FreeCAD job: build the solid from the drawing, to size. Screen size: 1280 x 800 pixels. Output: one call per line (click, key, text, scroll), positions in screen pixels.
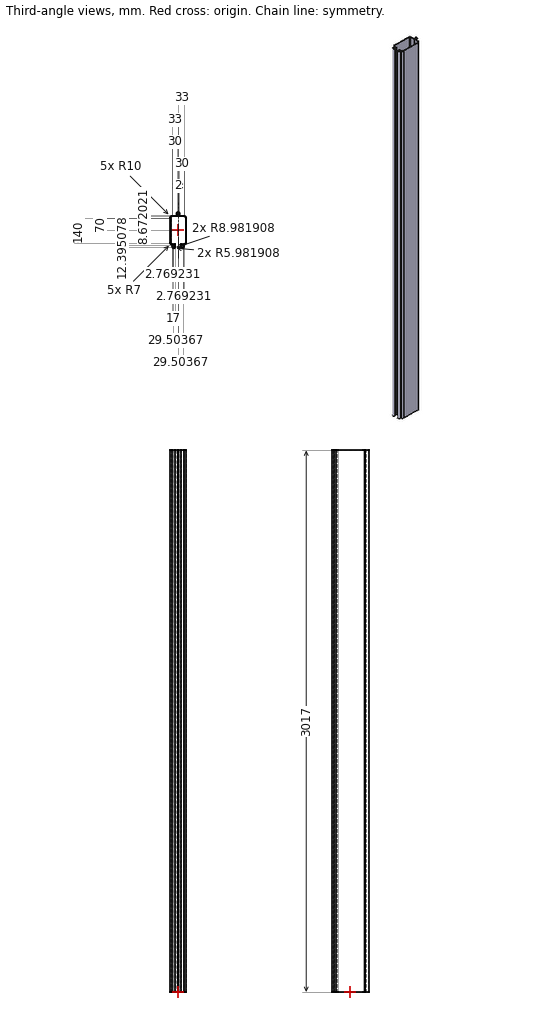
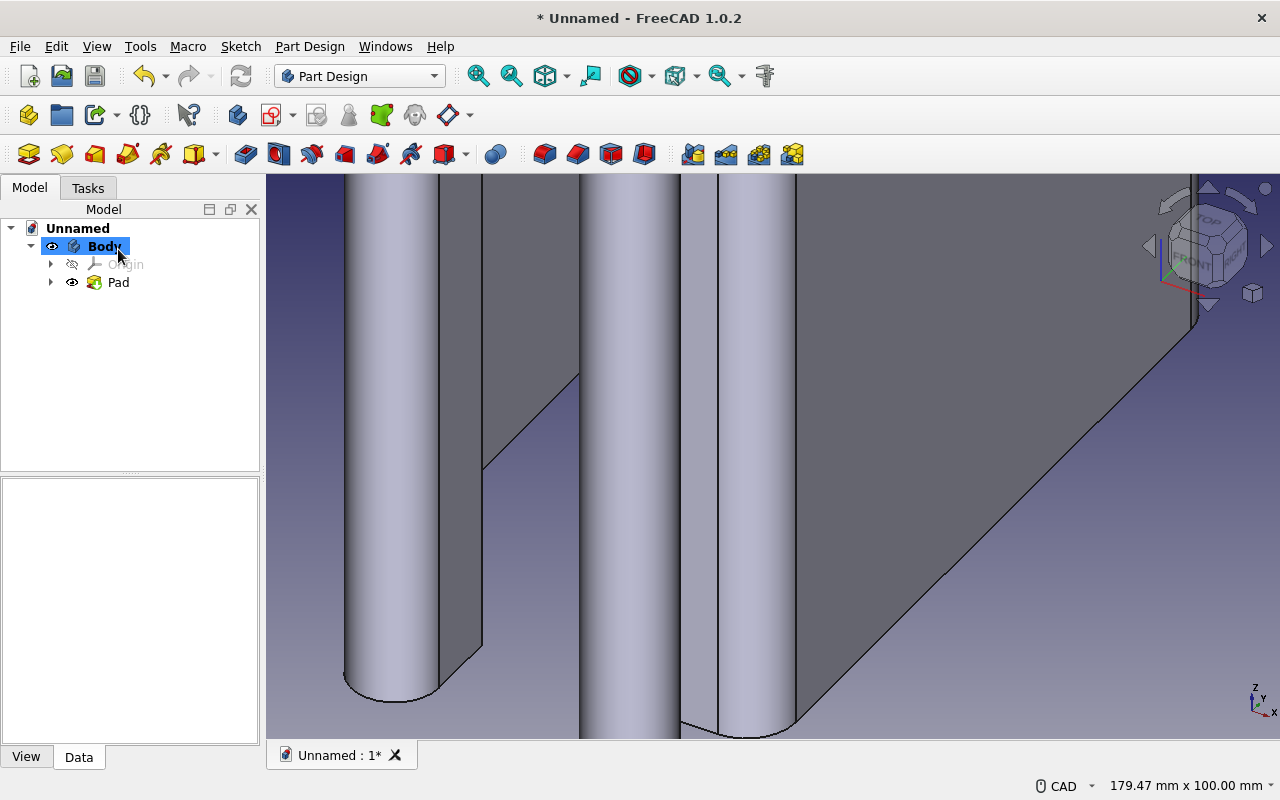
key(0)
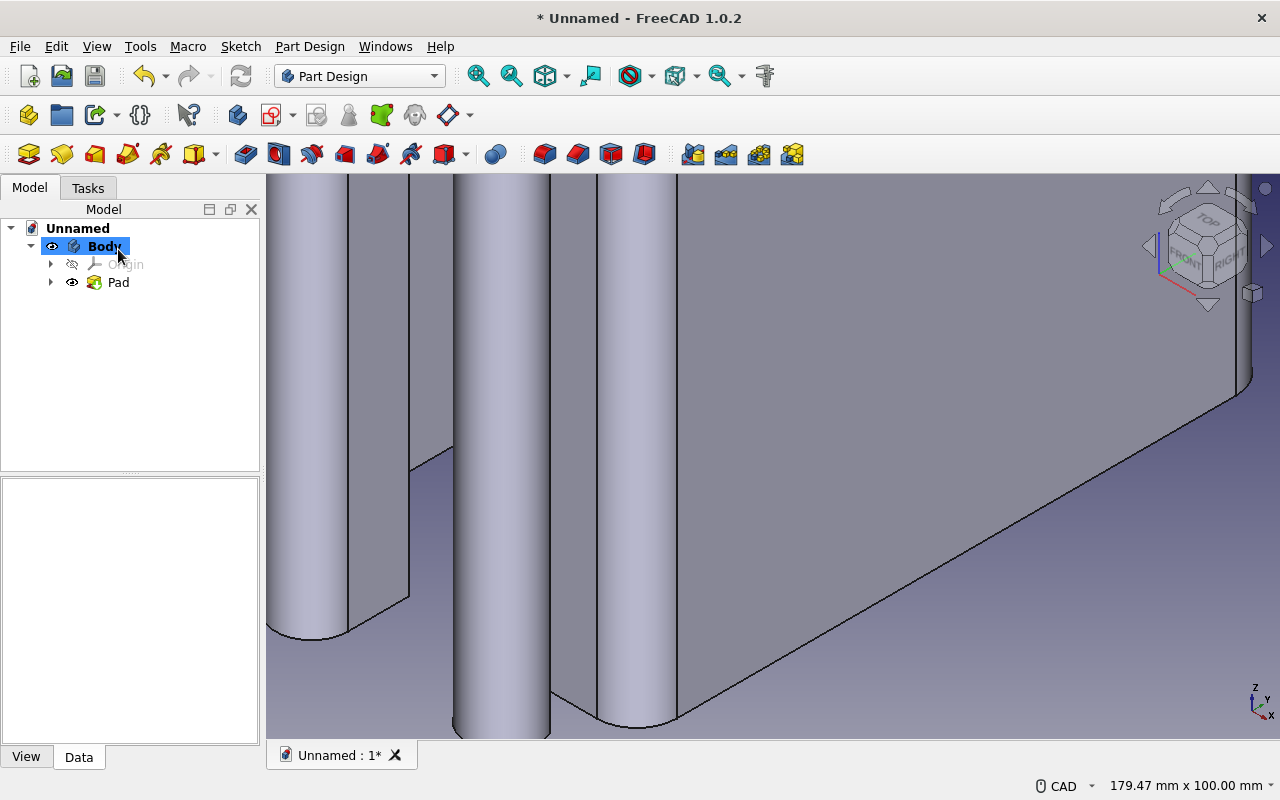
click(479, 76)